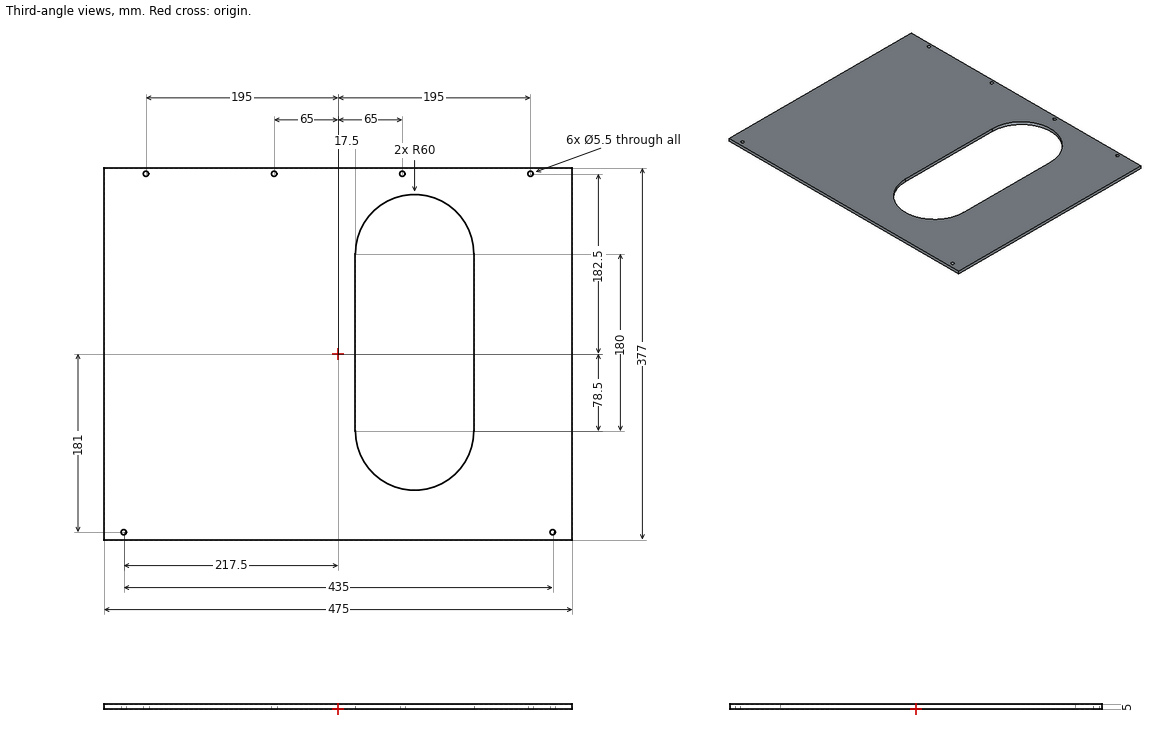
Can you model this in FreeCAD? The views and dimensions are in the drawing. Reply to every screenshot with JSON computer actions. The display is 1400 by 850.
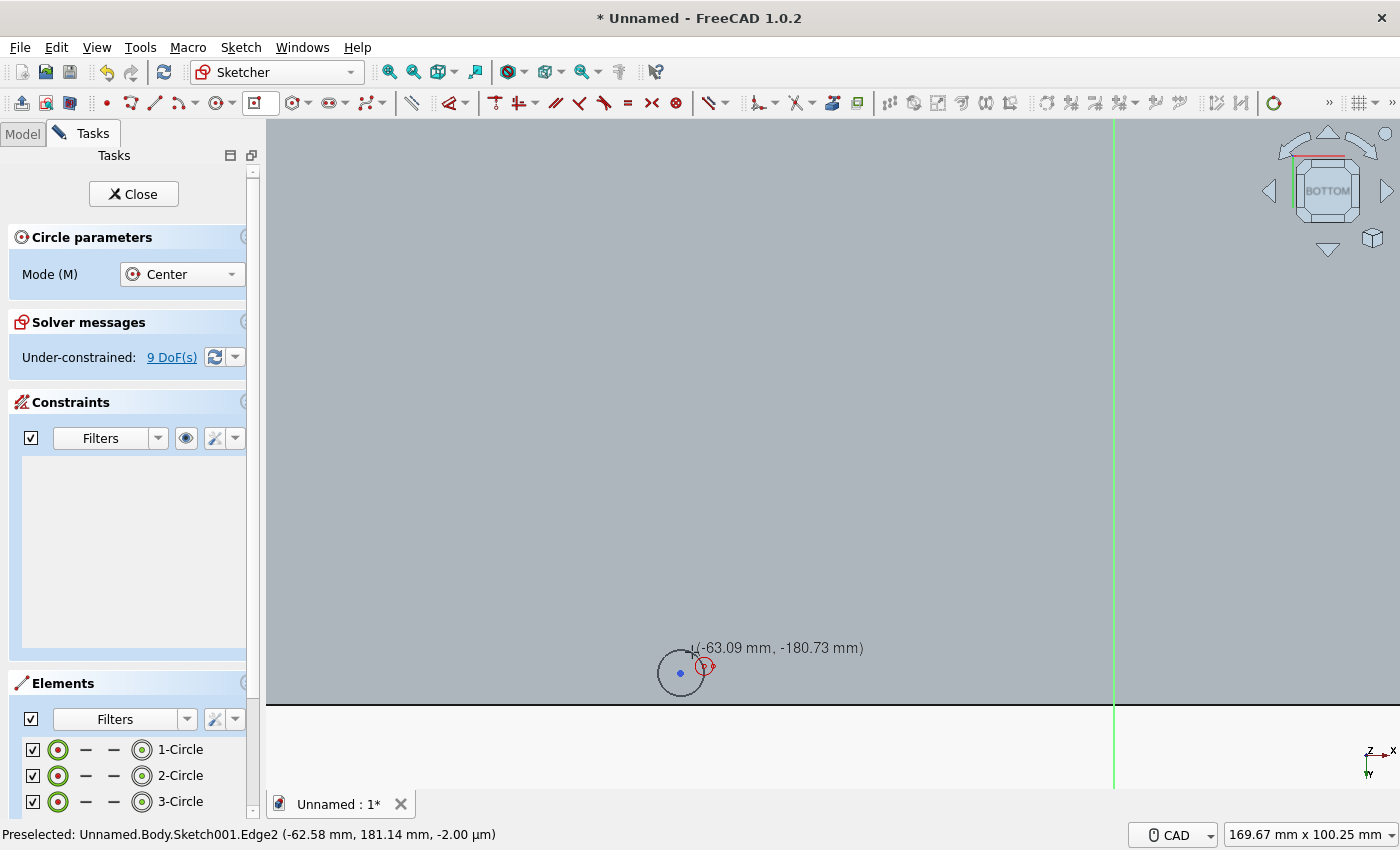
{"action": "scroll", "coordinate": [695, 653], "scroll_direction": "down", "scroll_amount": 9}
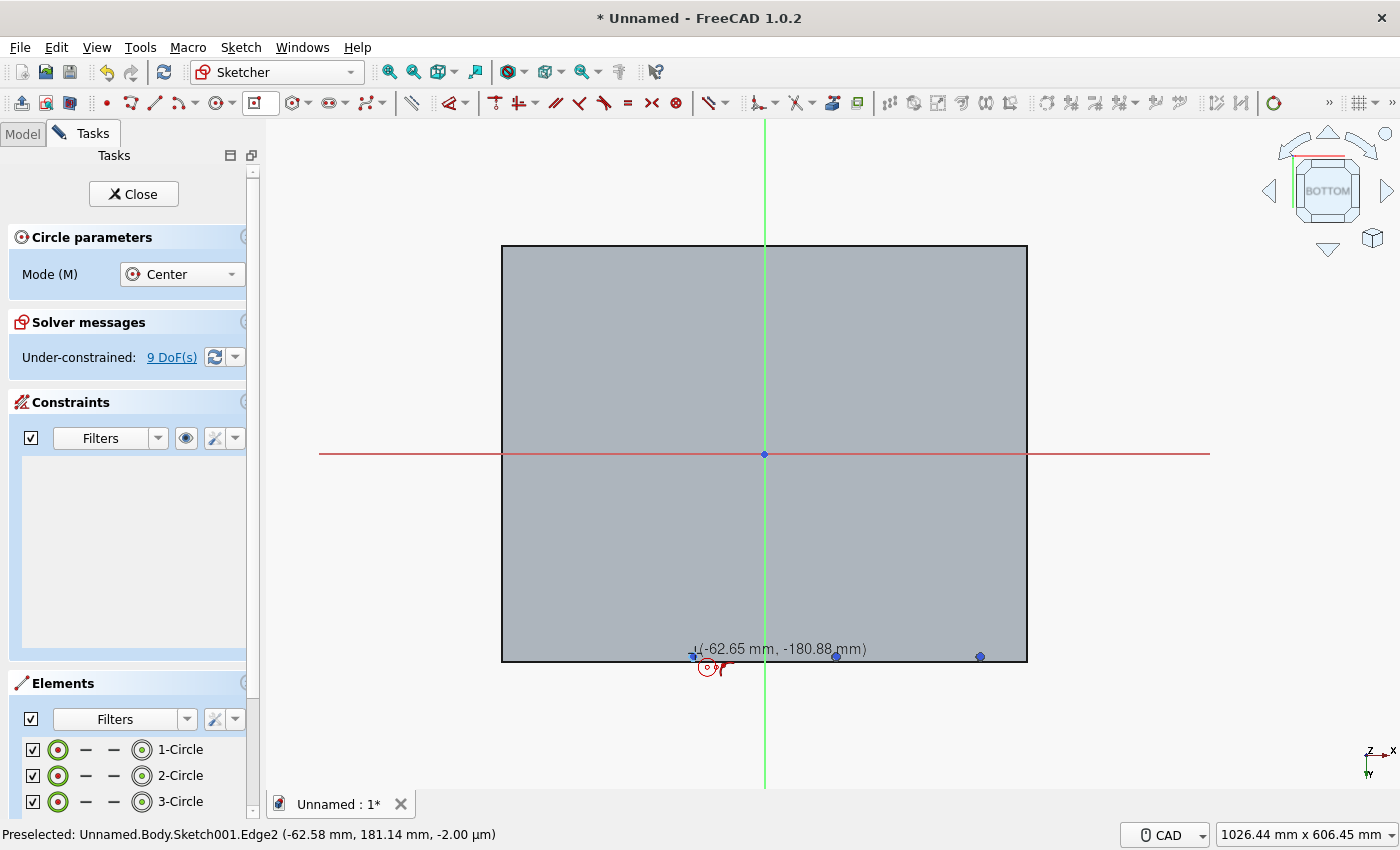
{"action": "scroll", "coordinate": [549, 656], "scroll_direction": "up", "scroll_amount": 11}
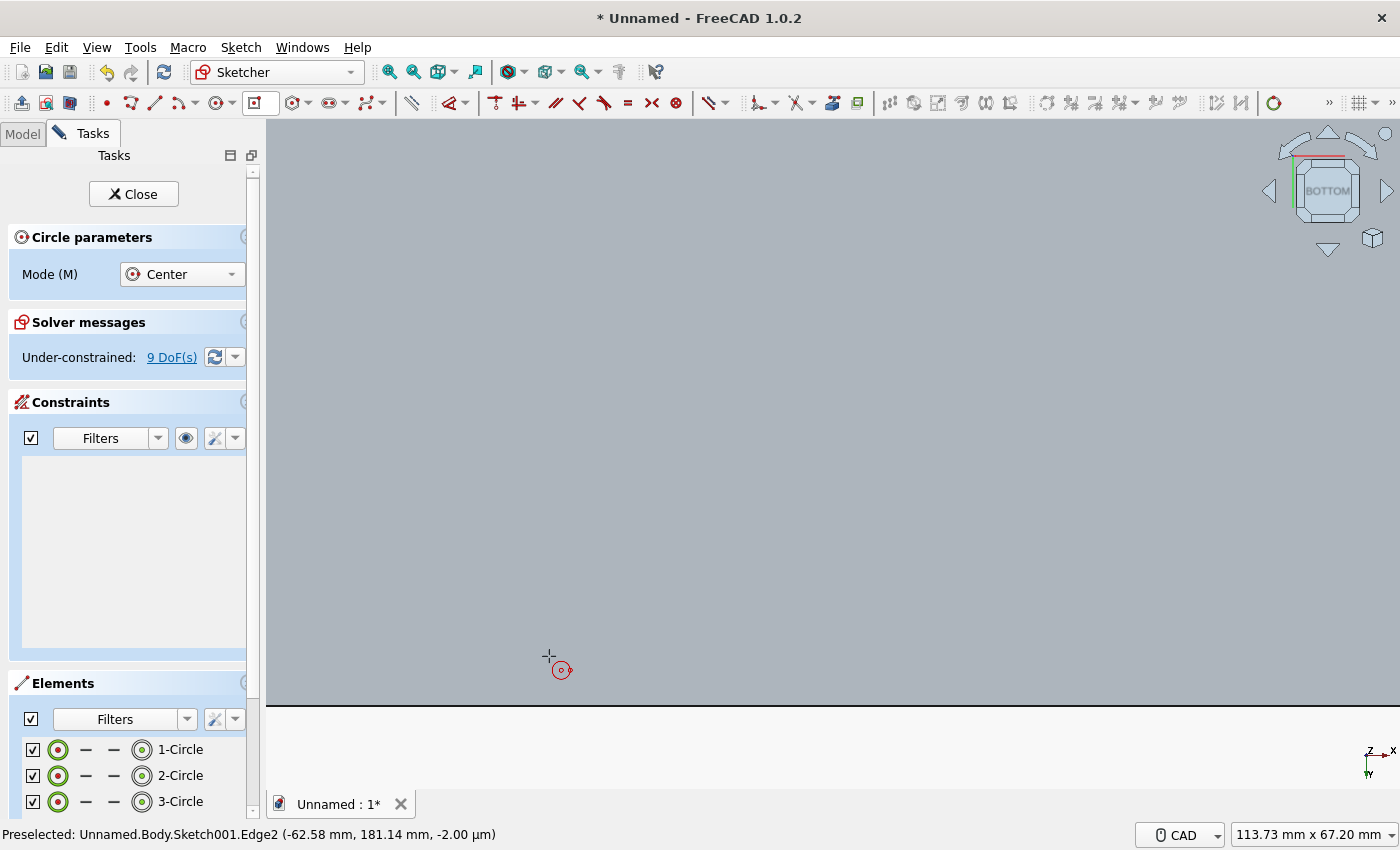
{"action": "scroll", "coordinate": [549, 656], "scroll_direction": "down", "scroll_amount": 11}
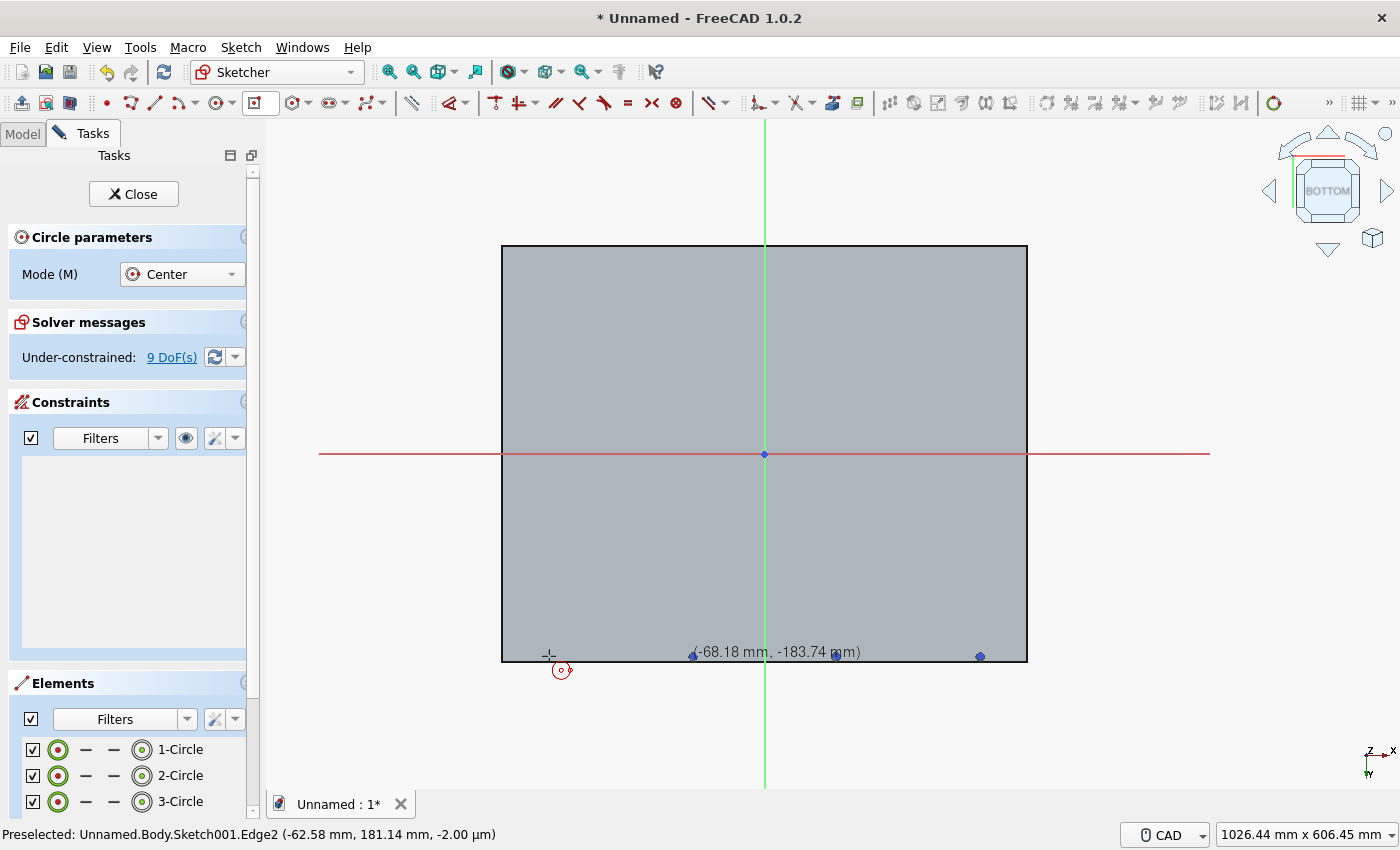
{"action": "left_click", "coordinate": [549, 656]}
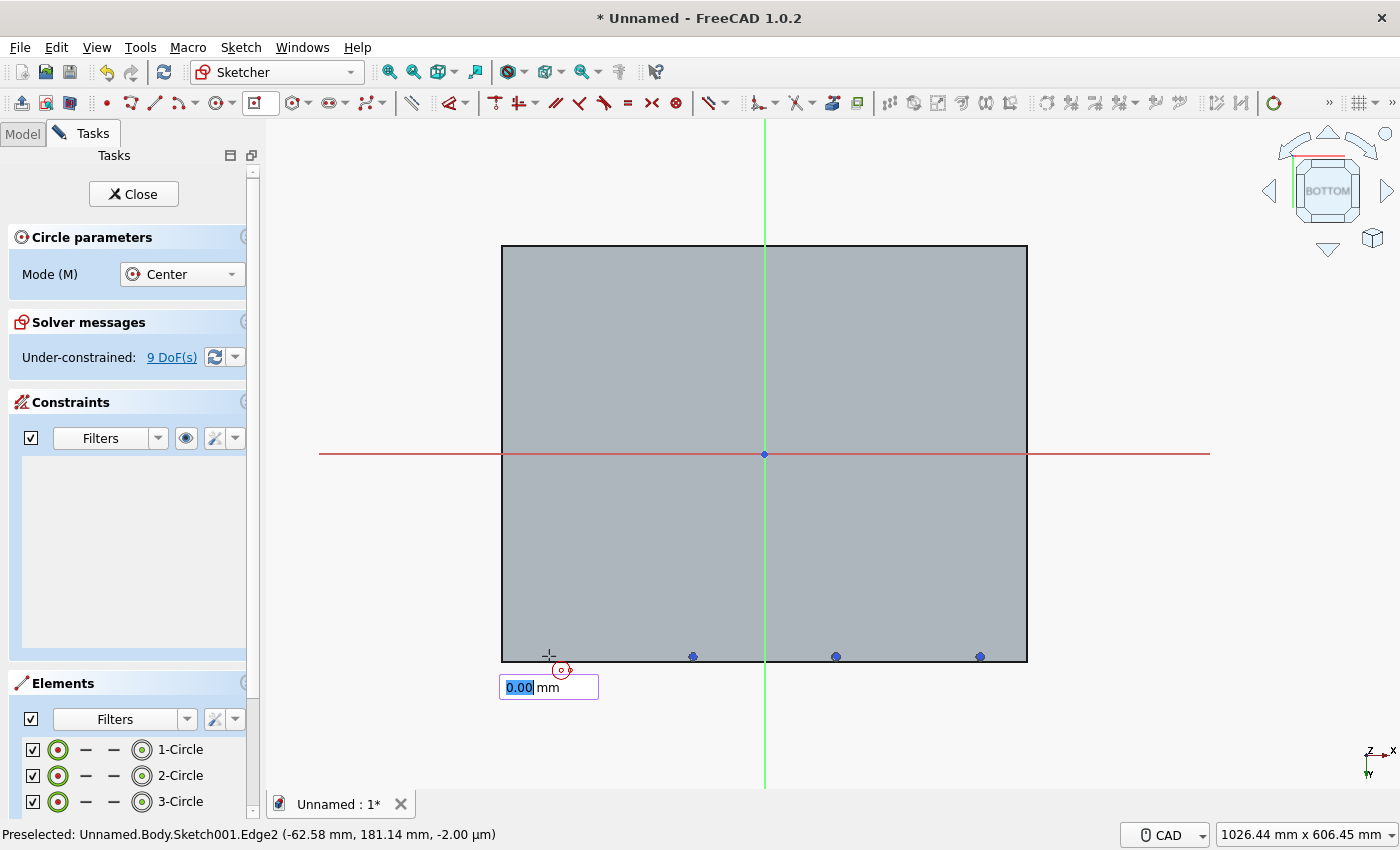
{"action": "scroll", "coordinate": [551, 653], "scroll_direction": "up", "scroll_amount": 9}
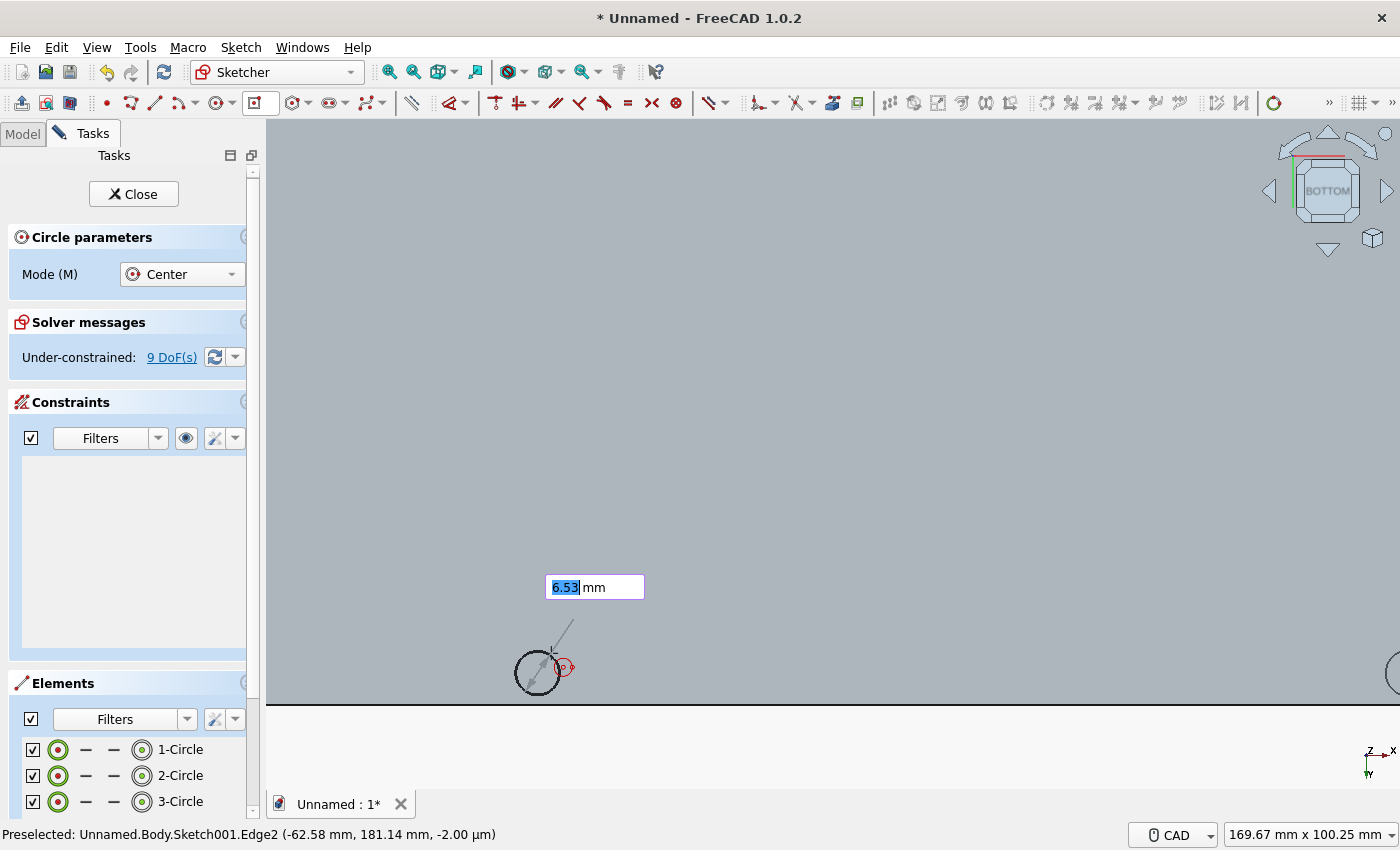
{"action": "left_click", "coordinate": [551, 652]}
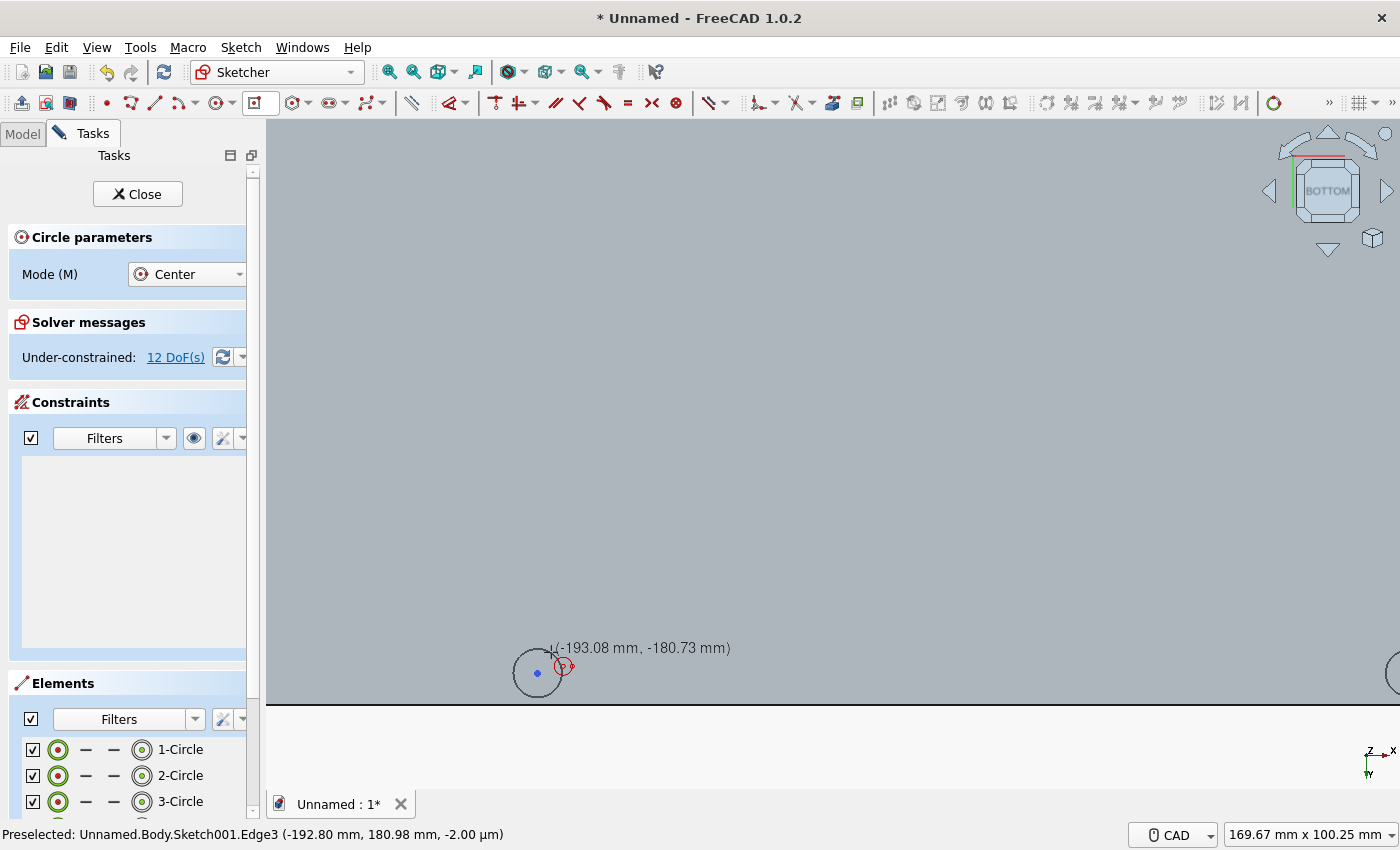
{"action": "scroll", "coordinate": [551, 653], "scroll_direction": "down", "scroll_amount": 9}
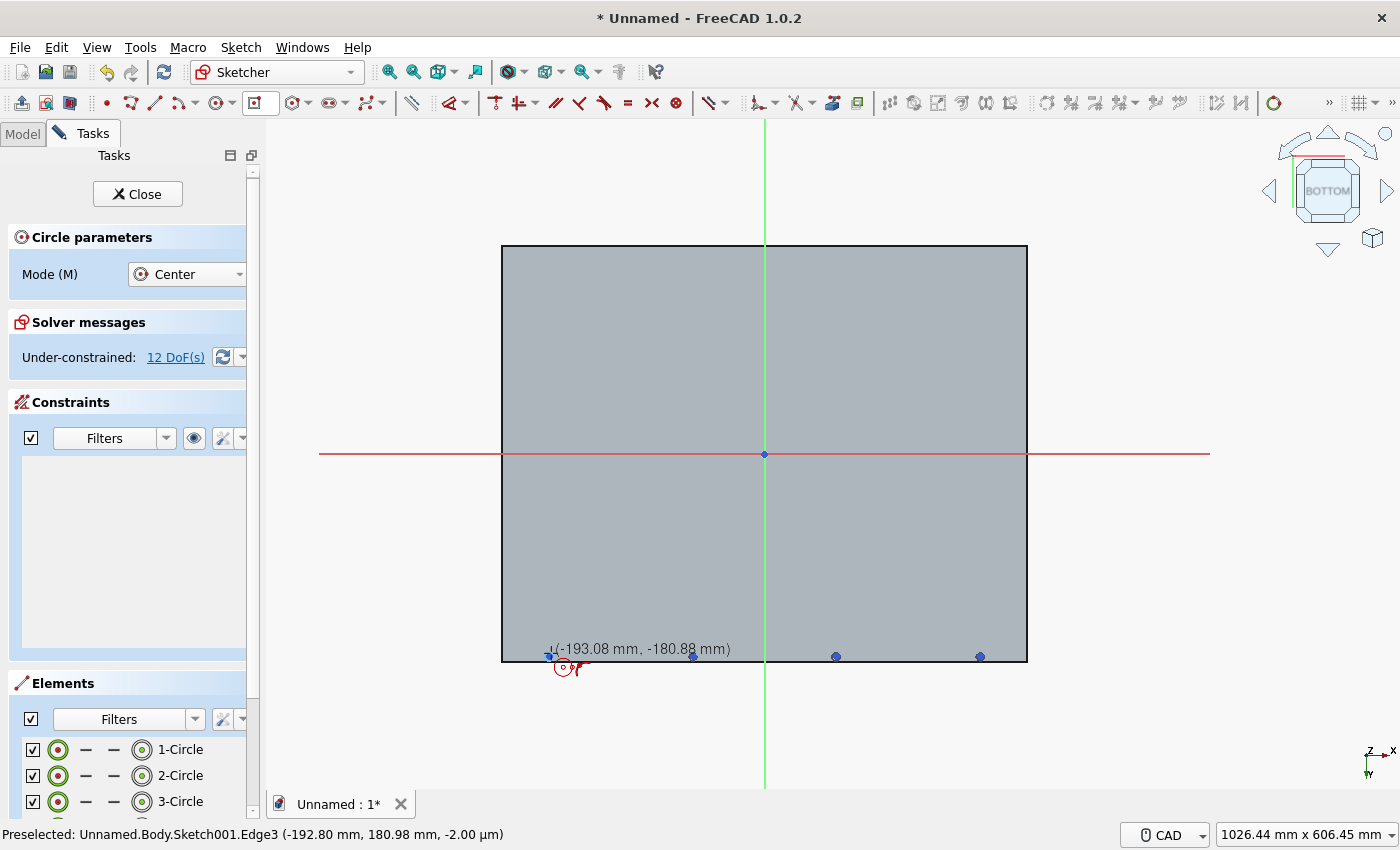
{"action": "scroll", "coordinate": [524, 254], "scroll_direction": "up", "scroll_amount": 11}